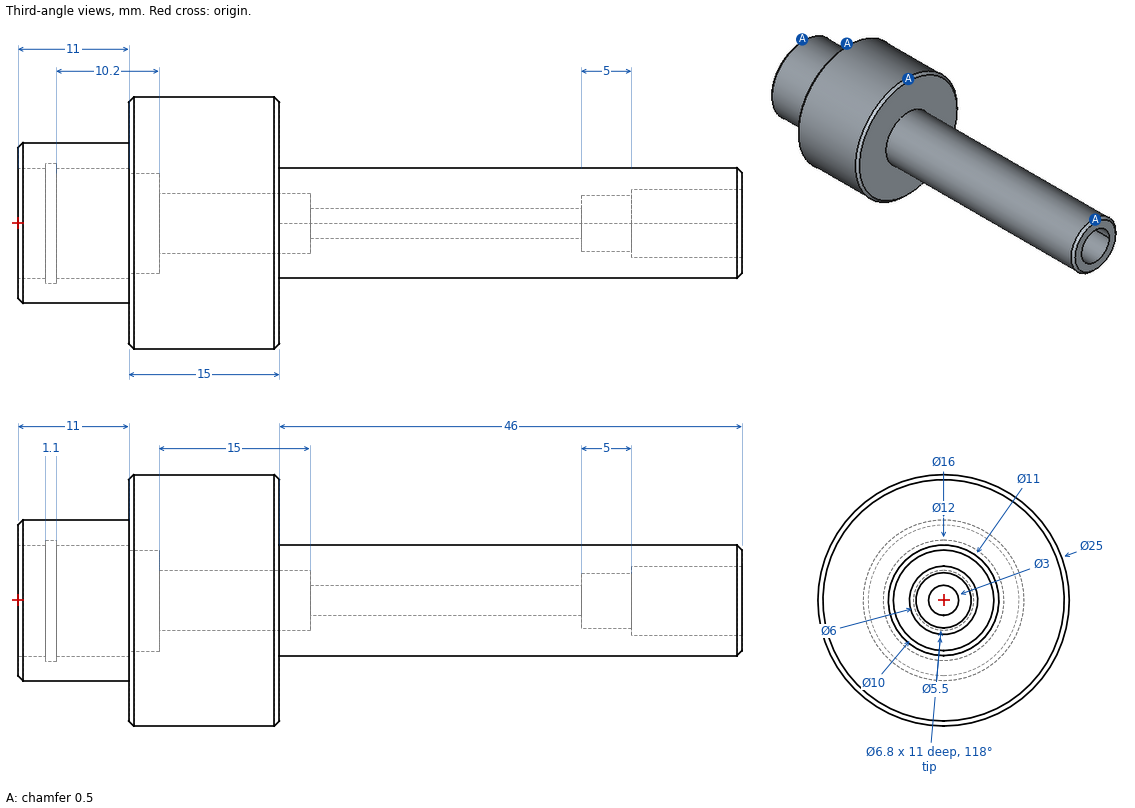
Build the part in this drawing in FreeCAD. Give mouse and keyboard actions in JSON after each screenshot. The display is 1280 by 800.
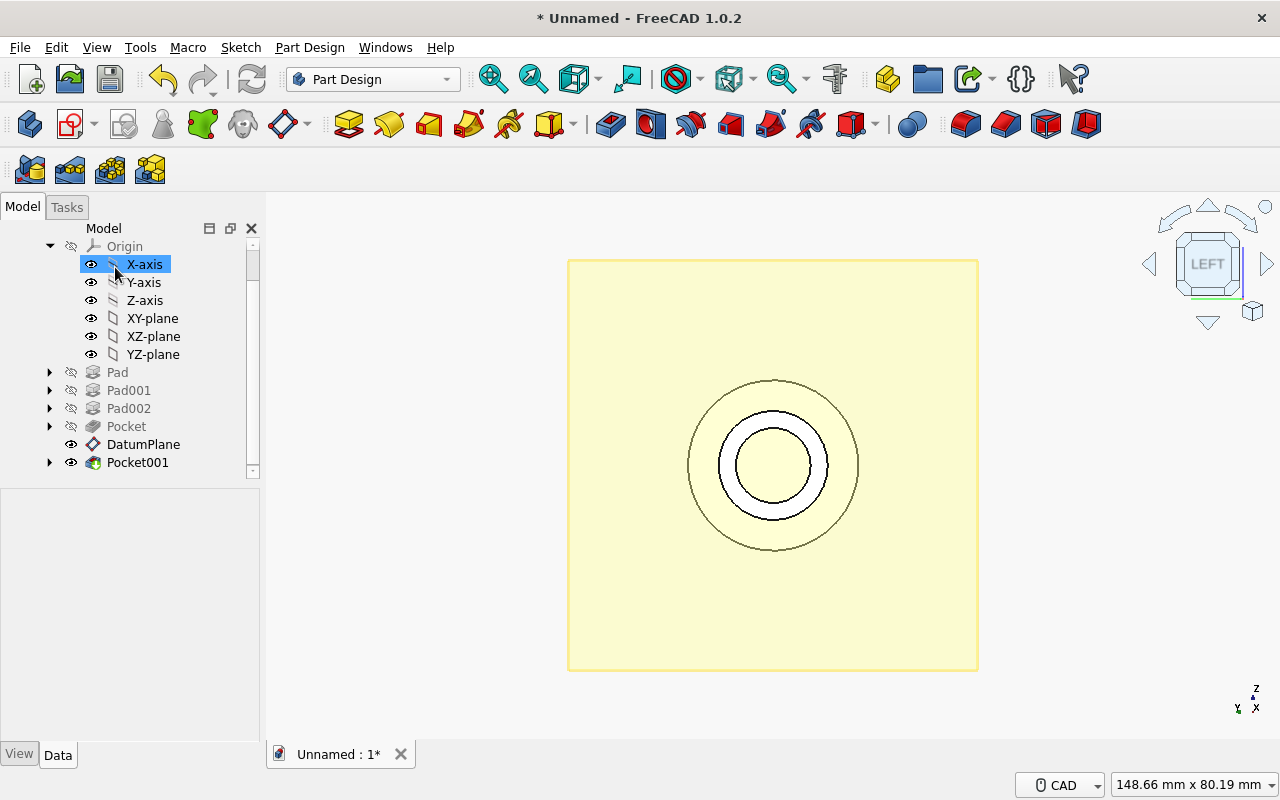
{"action": "left_click", "coordinate": [116, 444]}
{"action": "key", "text": "space"}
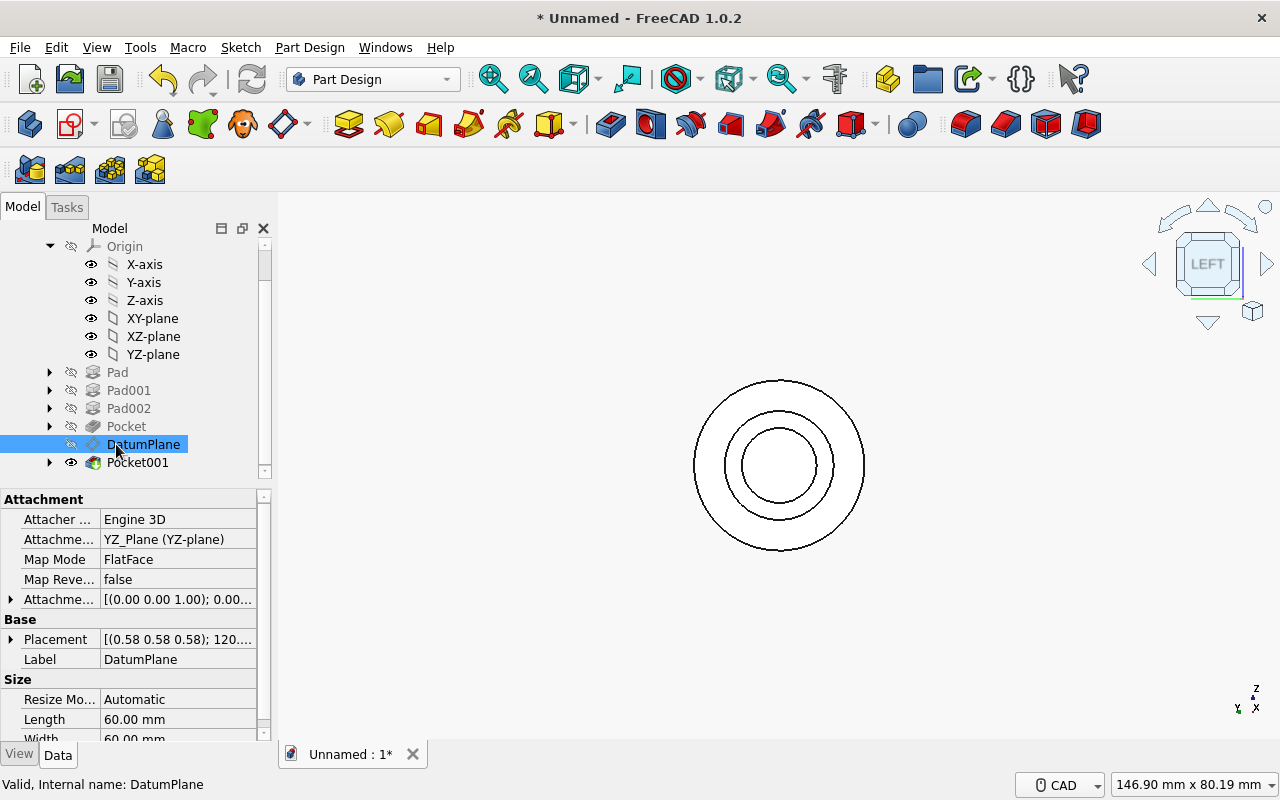
{"action": "left_click", "coordinate": [494, 80]}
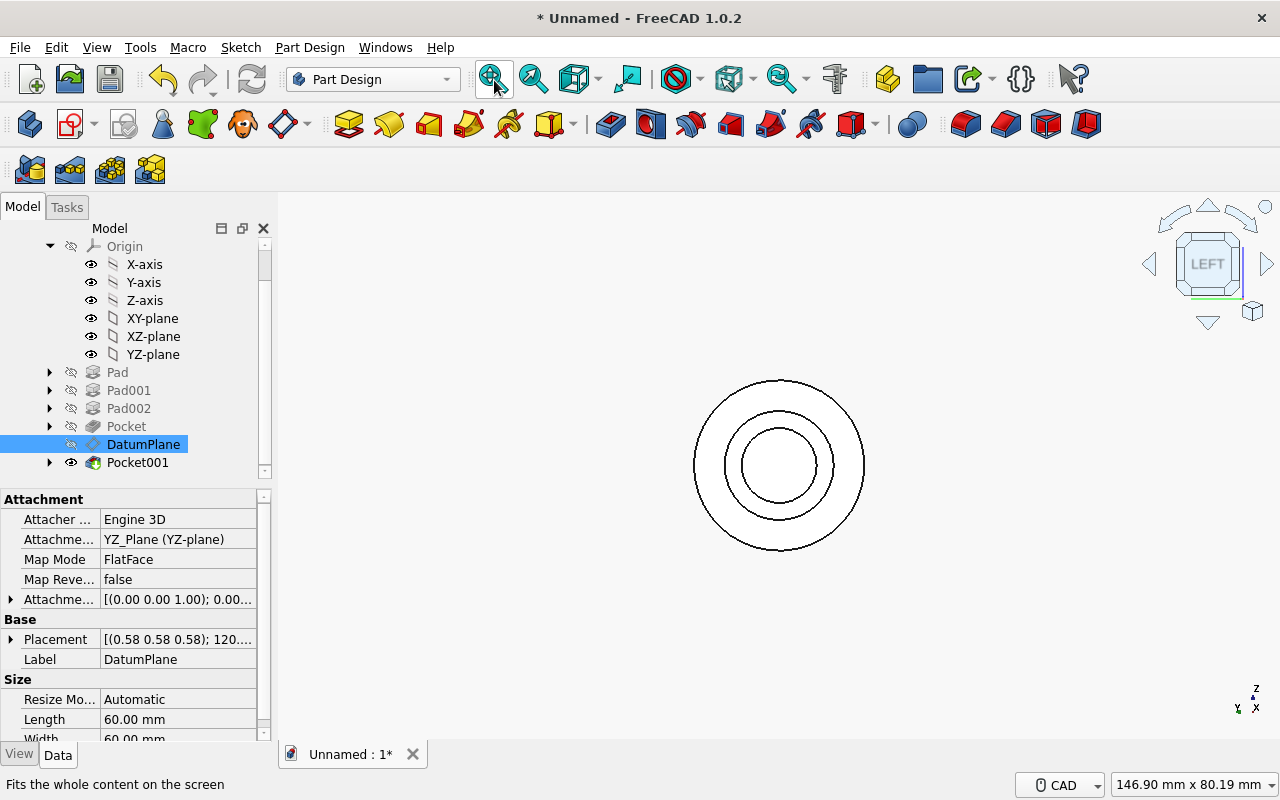
{"action": "left_click", "coordinate": [136, 354]}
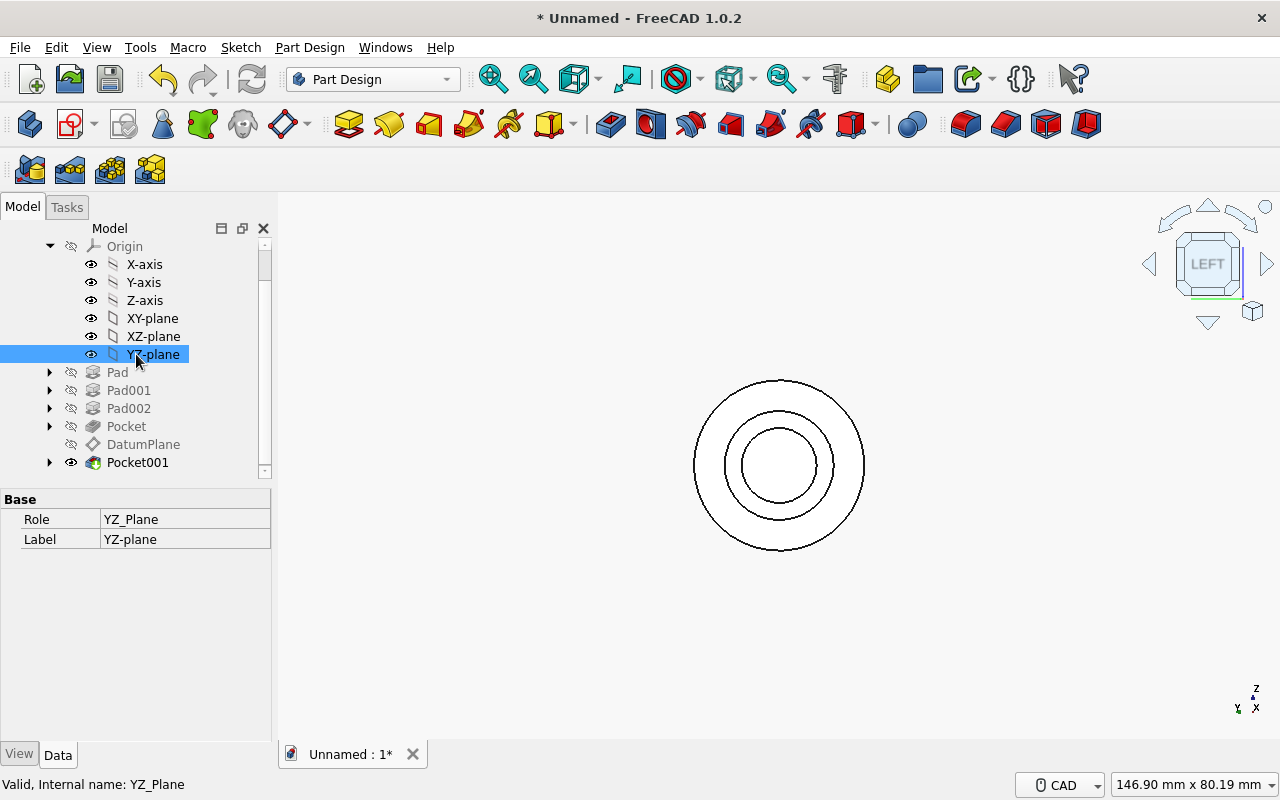
{"action": "left_click", "coordinate": [284, 124]}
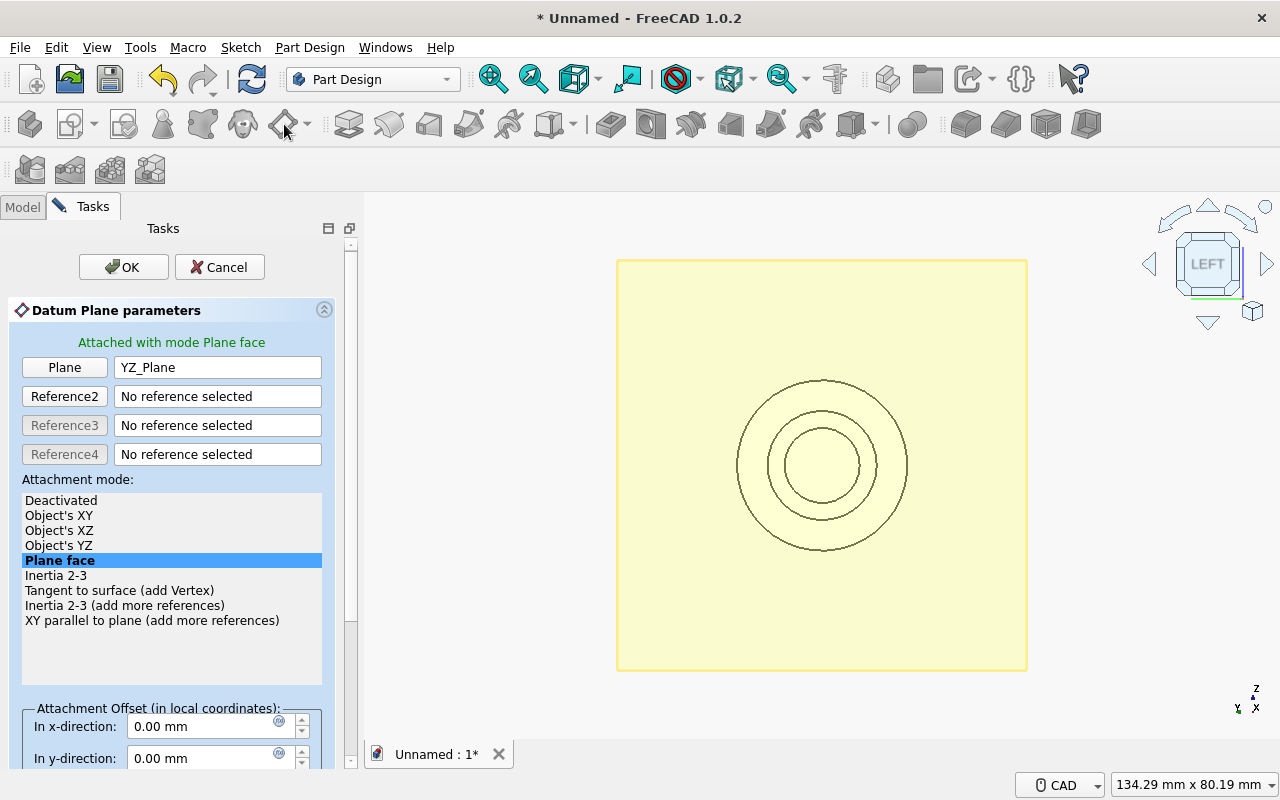
{"action": "scroll", "coordinate": [351, 503], "scroll_direction": "down", "scroll_amount": 2}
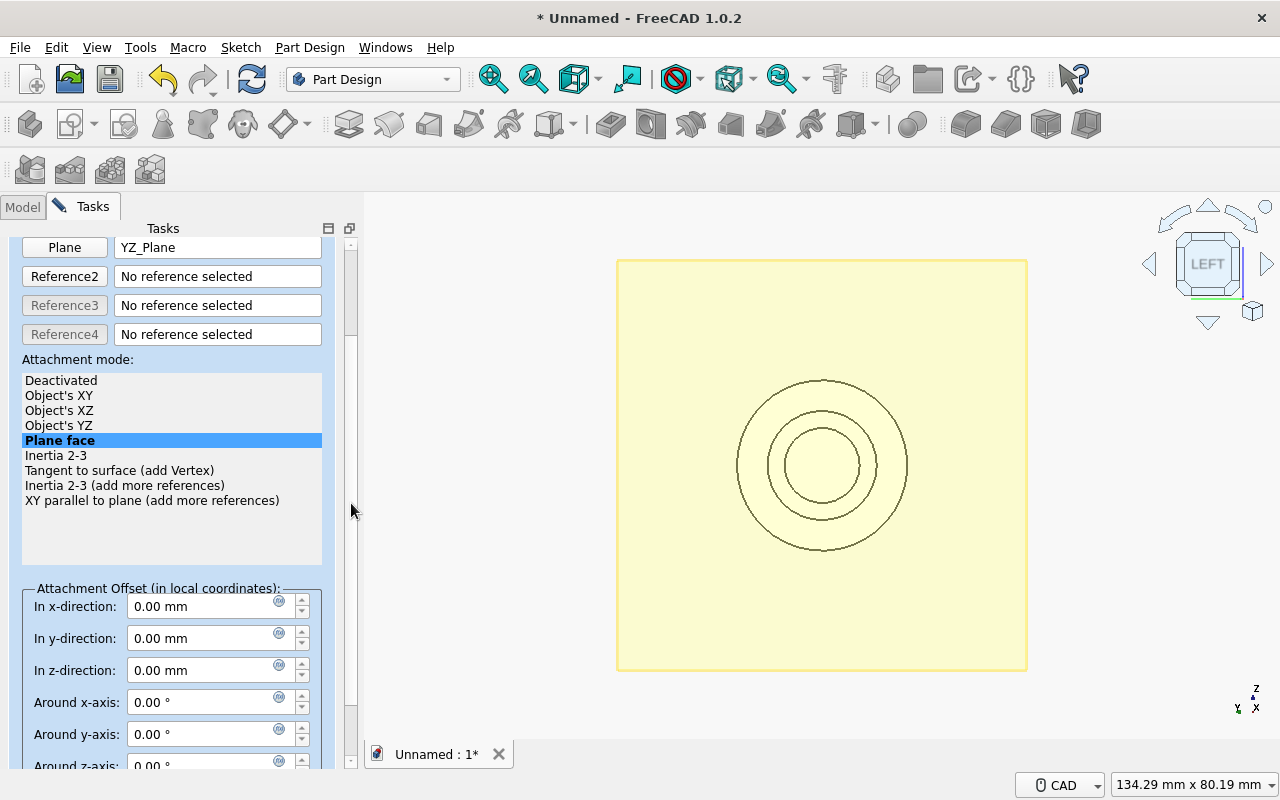
{"action": "triple_click", "coordinate": [210, 670]}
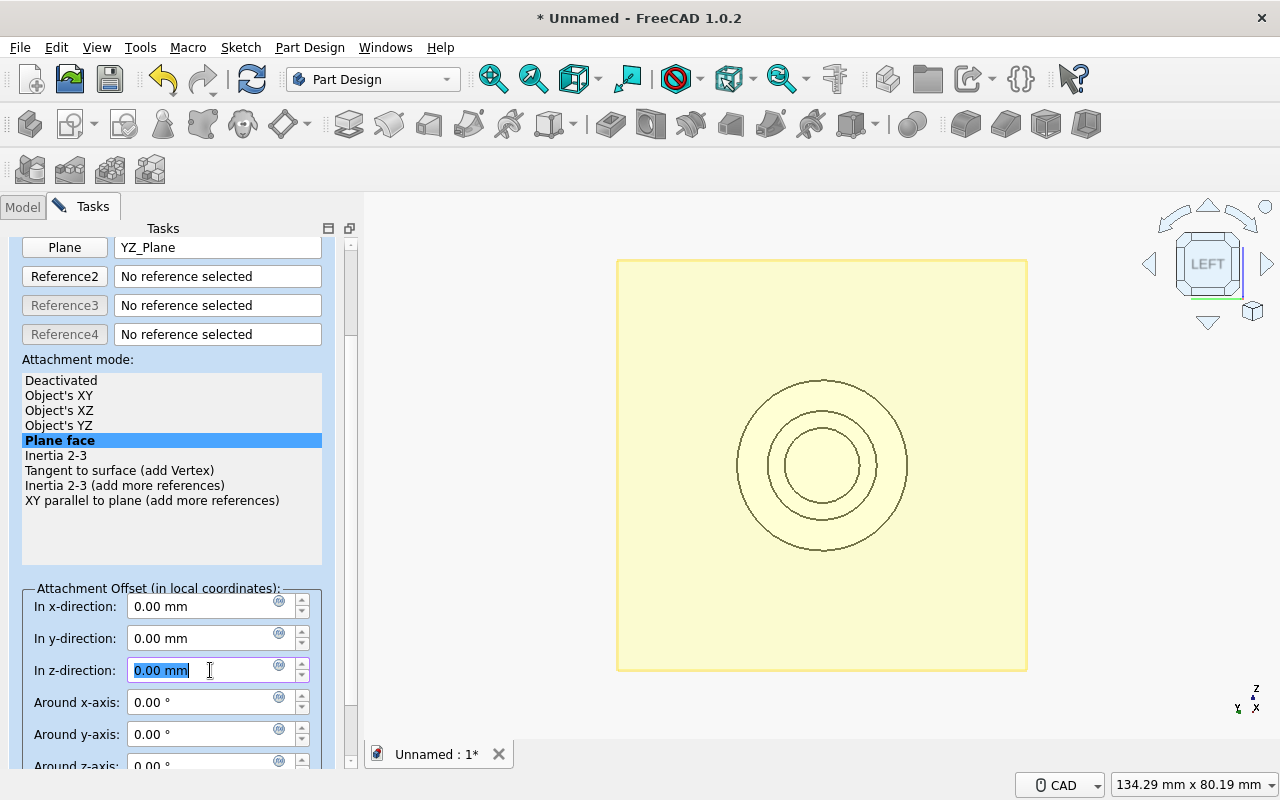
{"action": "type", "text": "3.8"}
{"action": "key", "text": "Tab"}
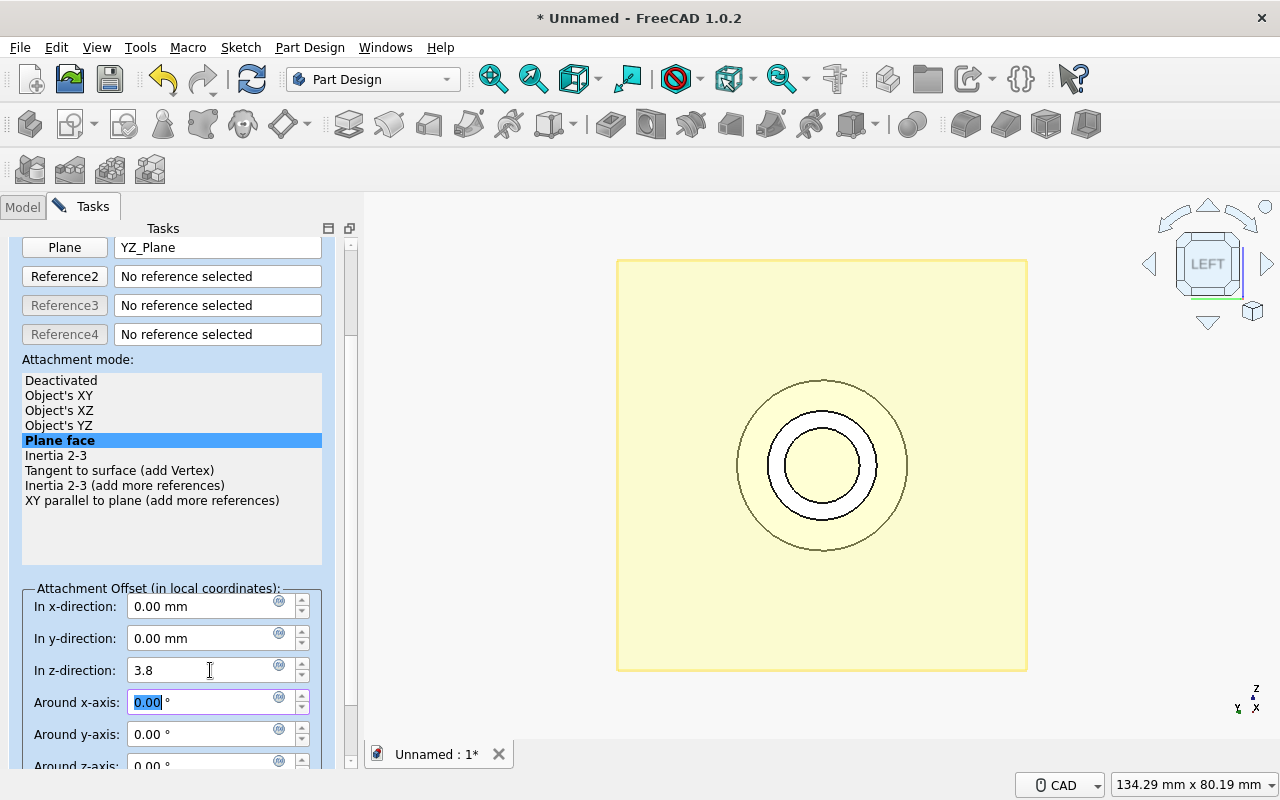
{"action": "scroll", "coordinate": [351, 503], "scroll_direction": "up", "scroll_amount": 3}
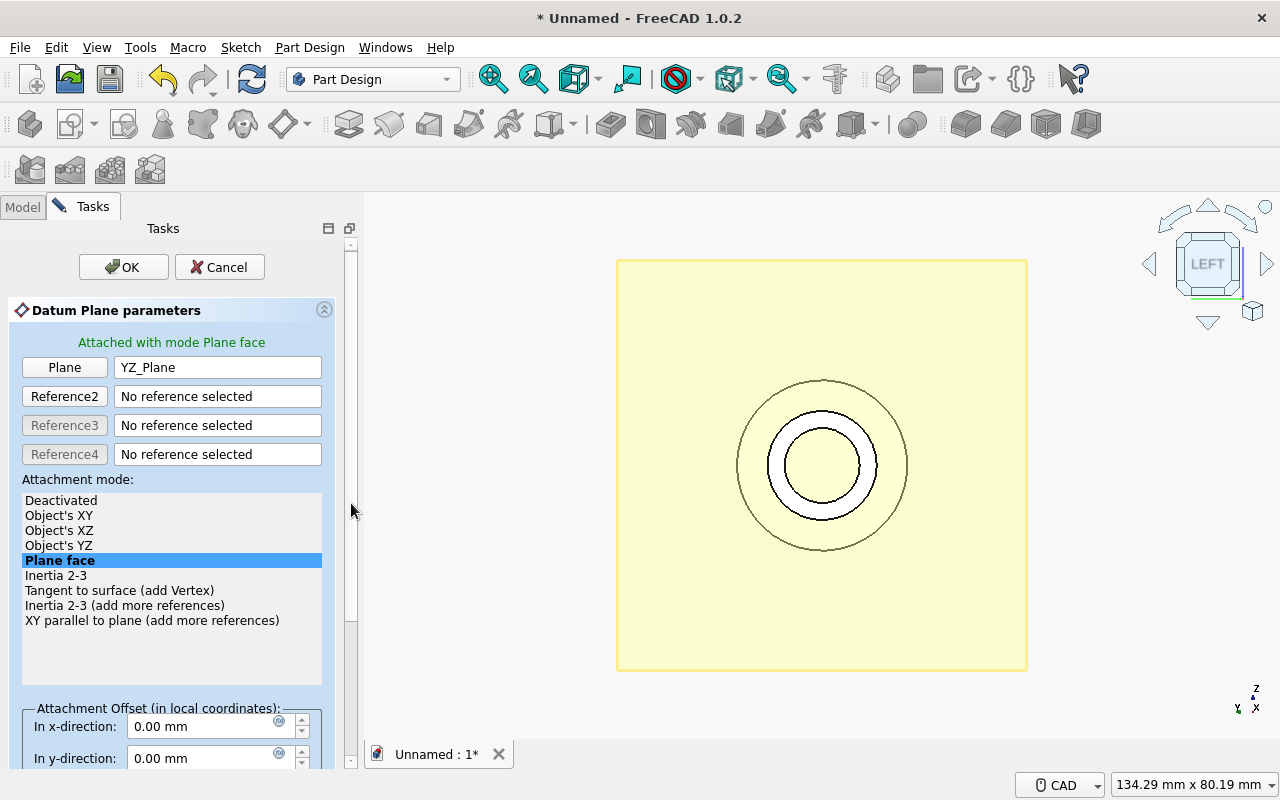
{"action": "left_click", "coordinate": [124, 267]}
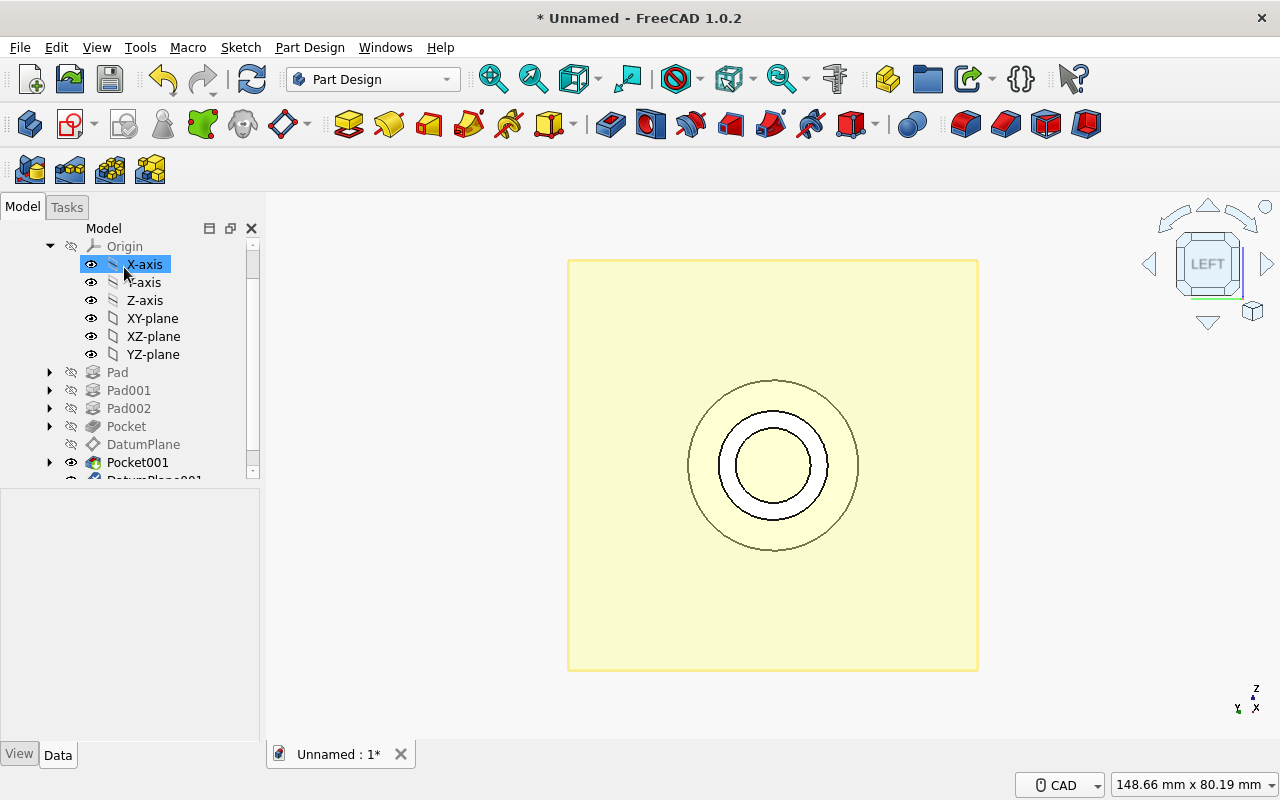
{"action": "scroll", "coordinate": [140, 350], "scroll_direction": "down", "scroll_amount": 3}